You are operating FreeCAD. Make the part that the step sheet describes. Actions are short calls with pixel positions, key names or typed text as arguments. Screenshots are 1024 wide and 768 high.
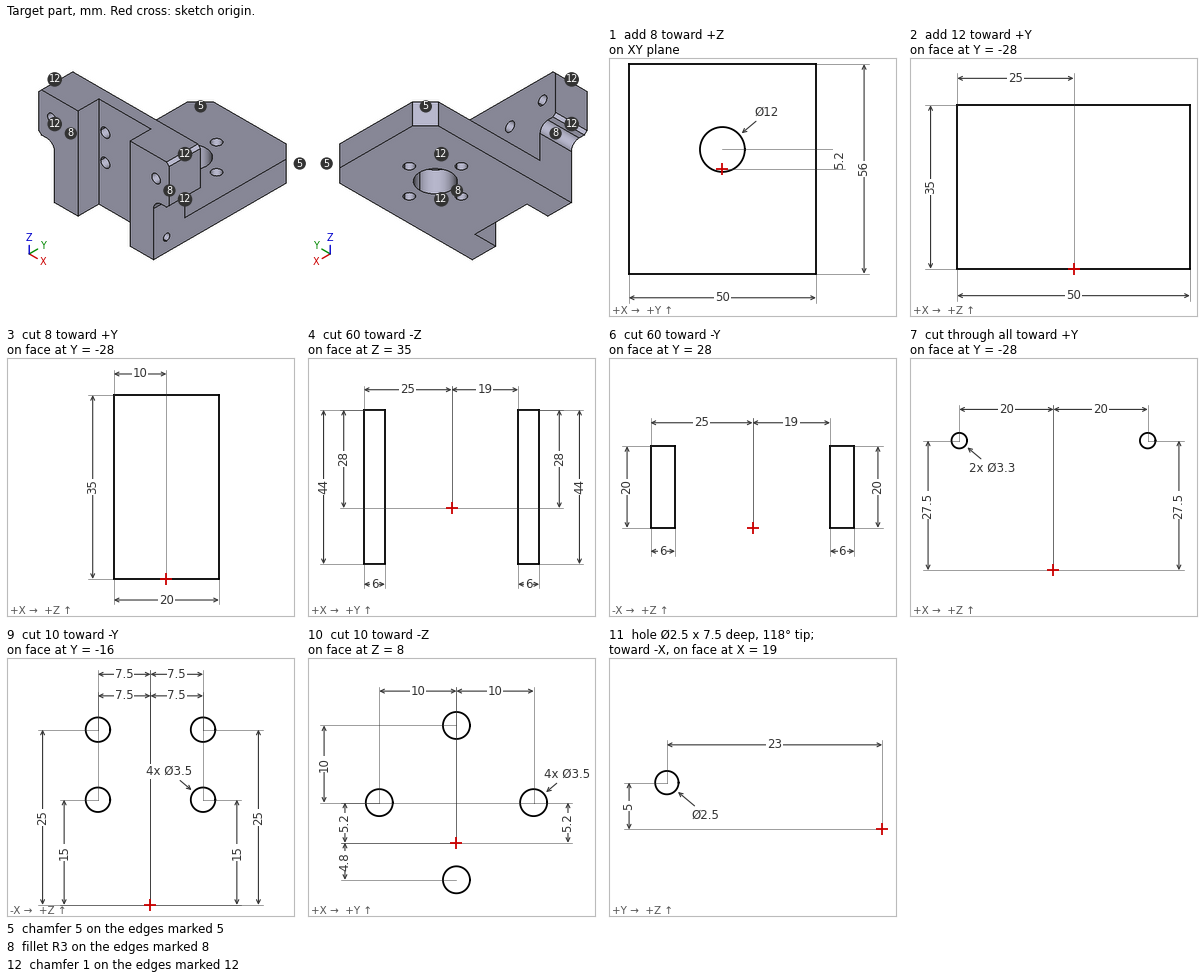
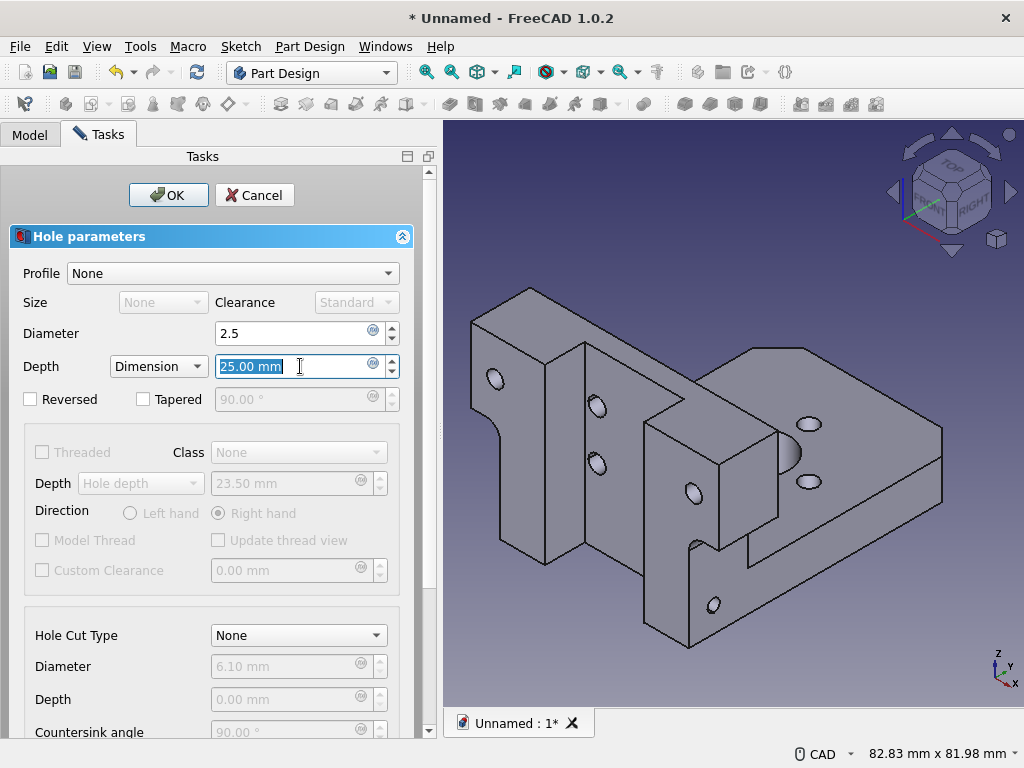
text(7.5)
key(Tab)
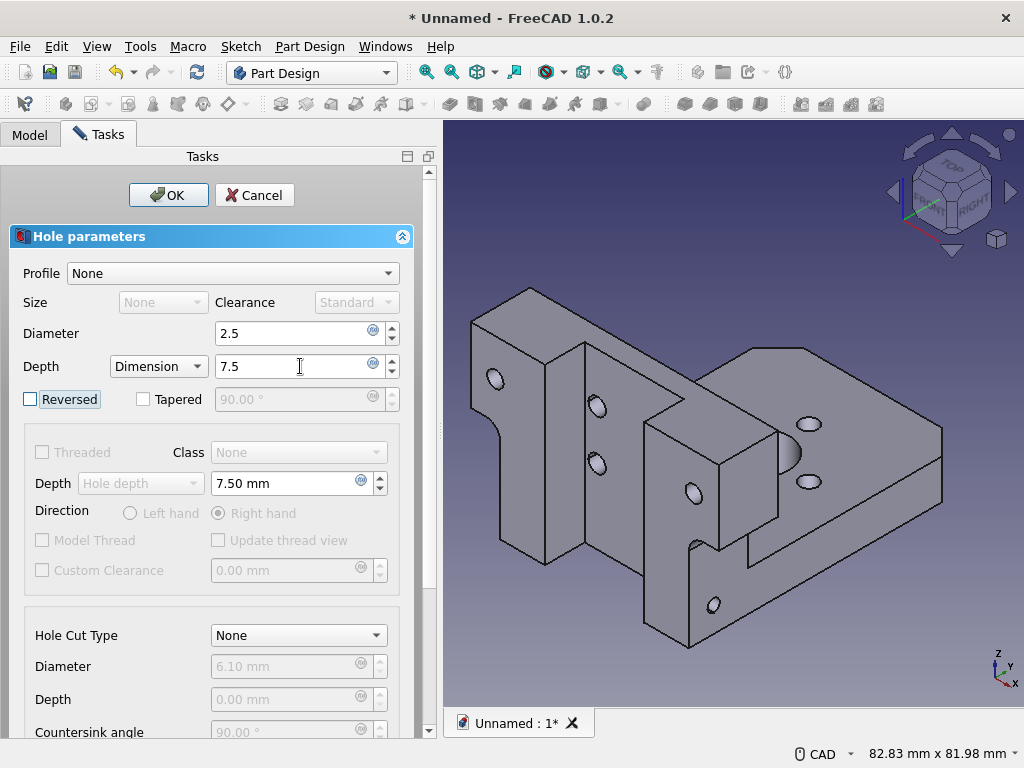
click(169, 195)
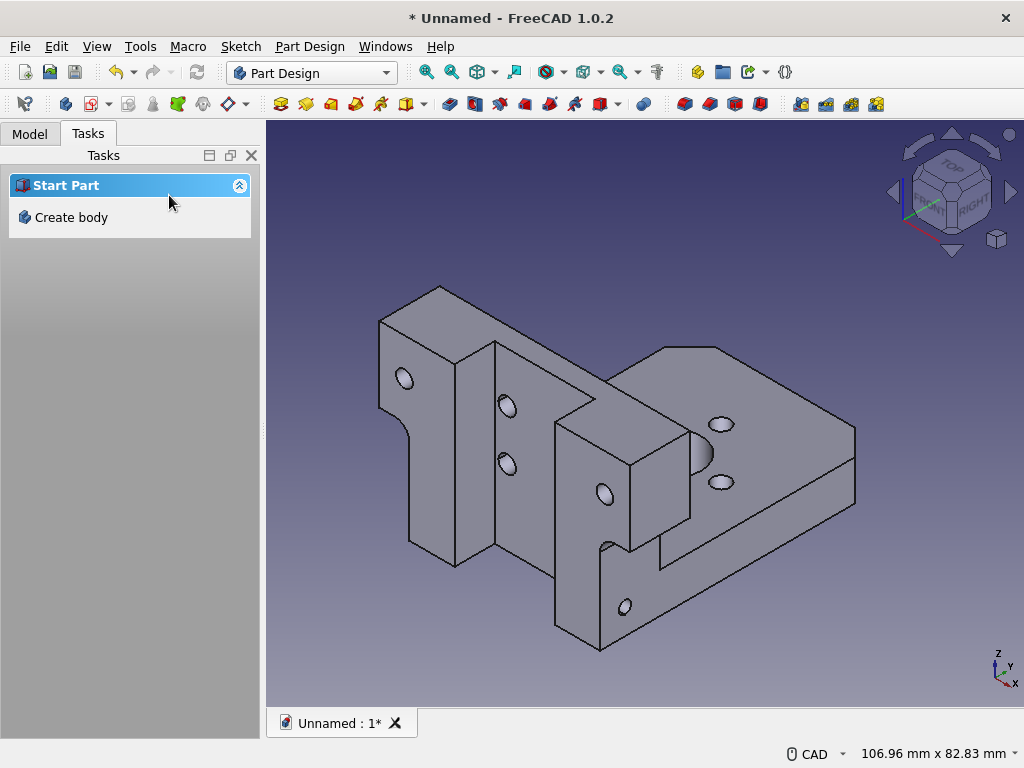
click(660, 447)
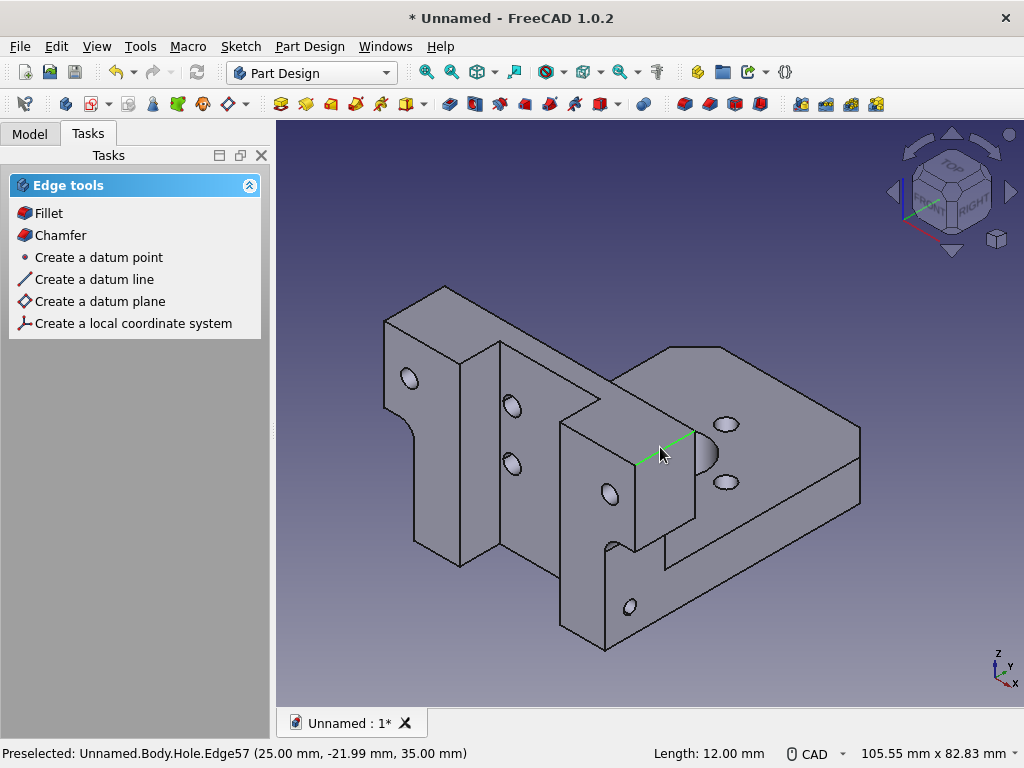
key(2)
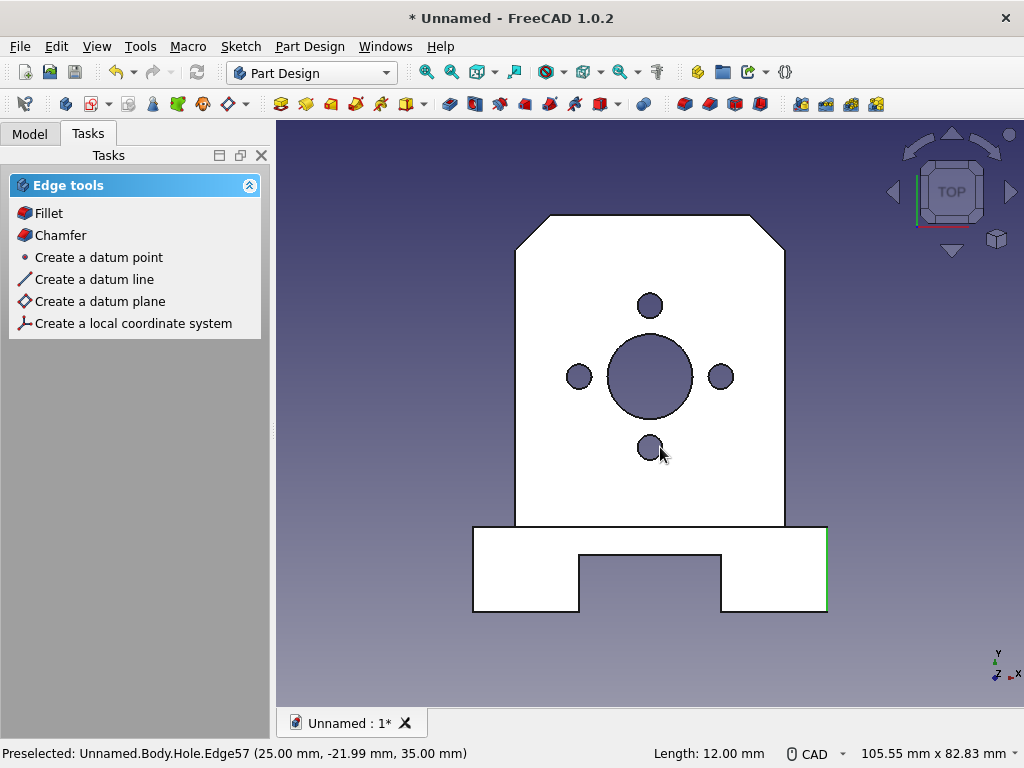
click(473, 568, ctrl)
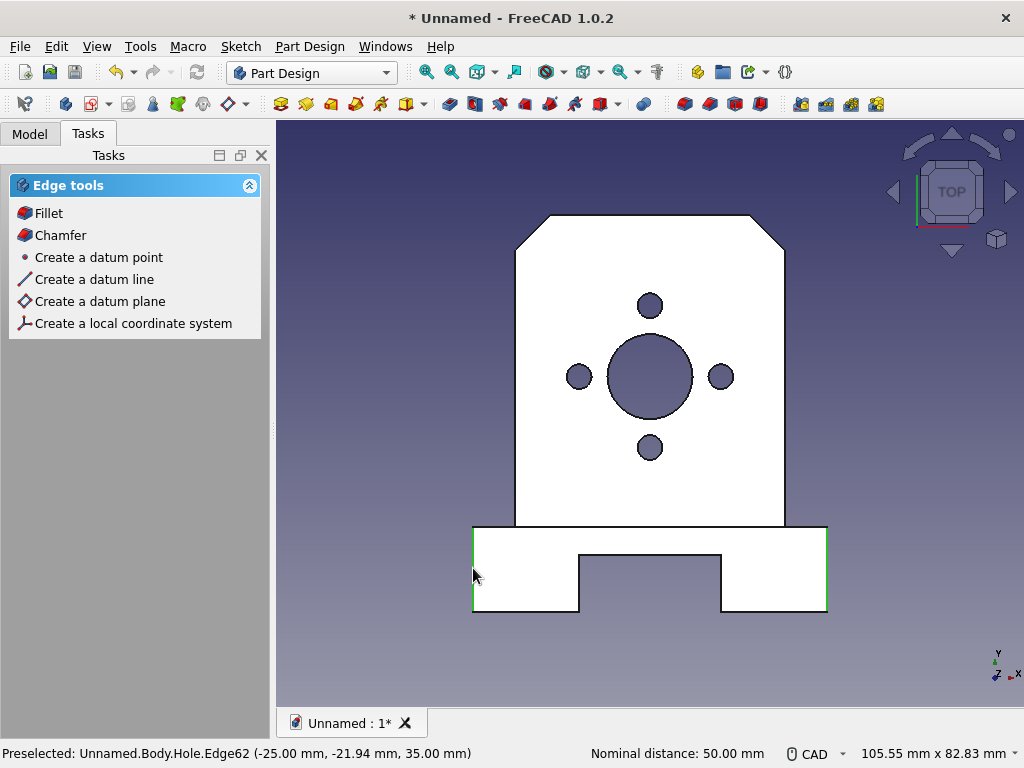
key(0)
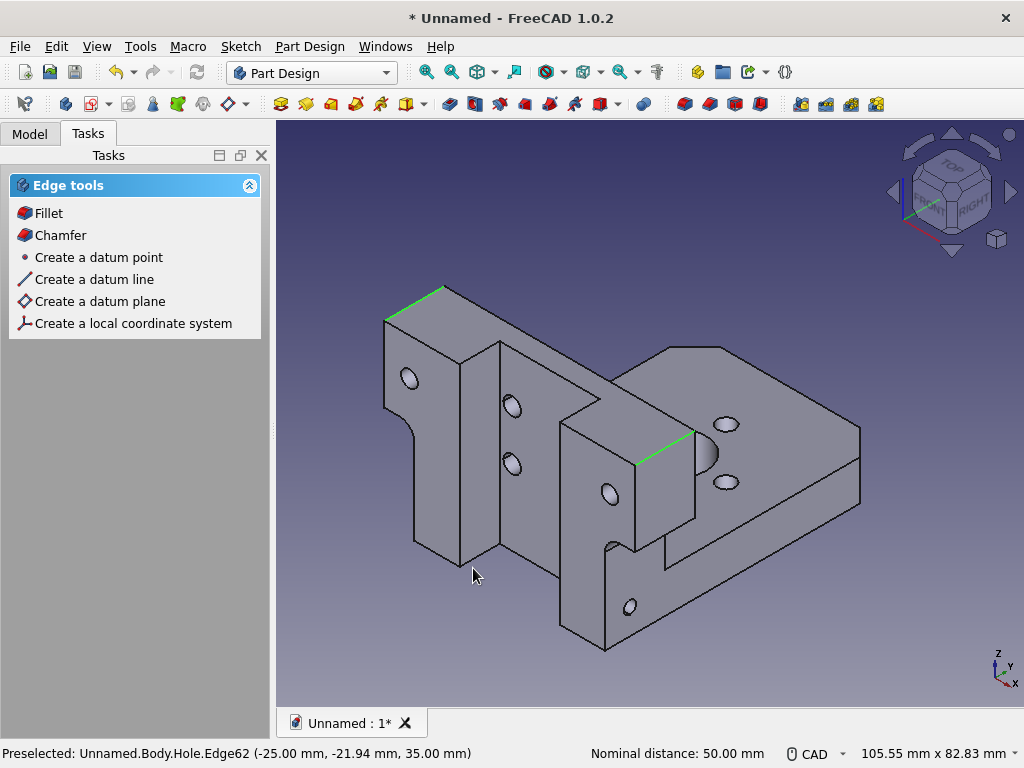
key(1)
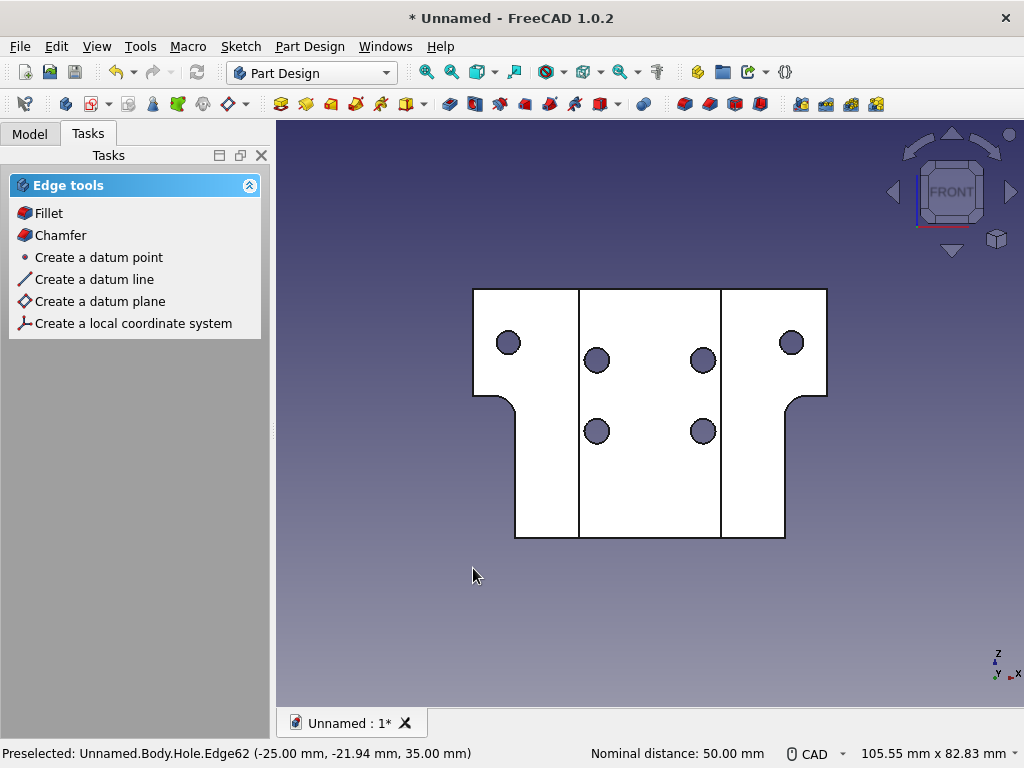
key(3)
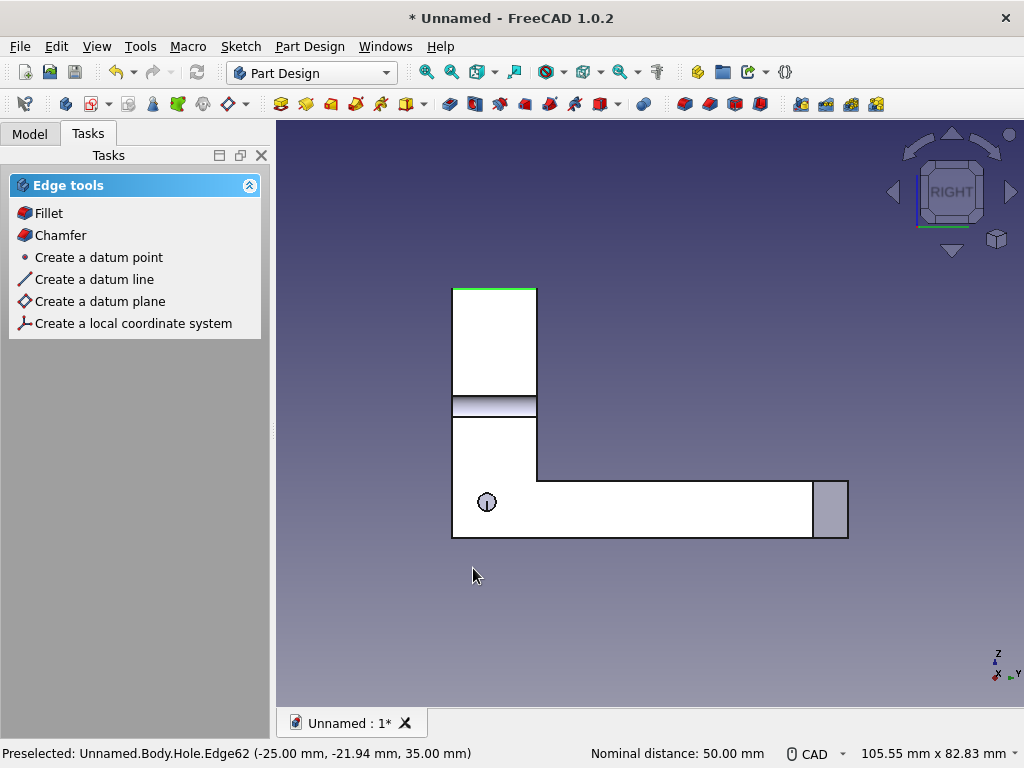
click(494, 395, ctrl)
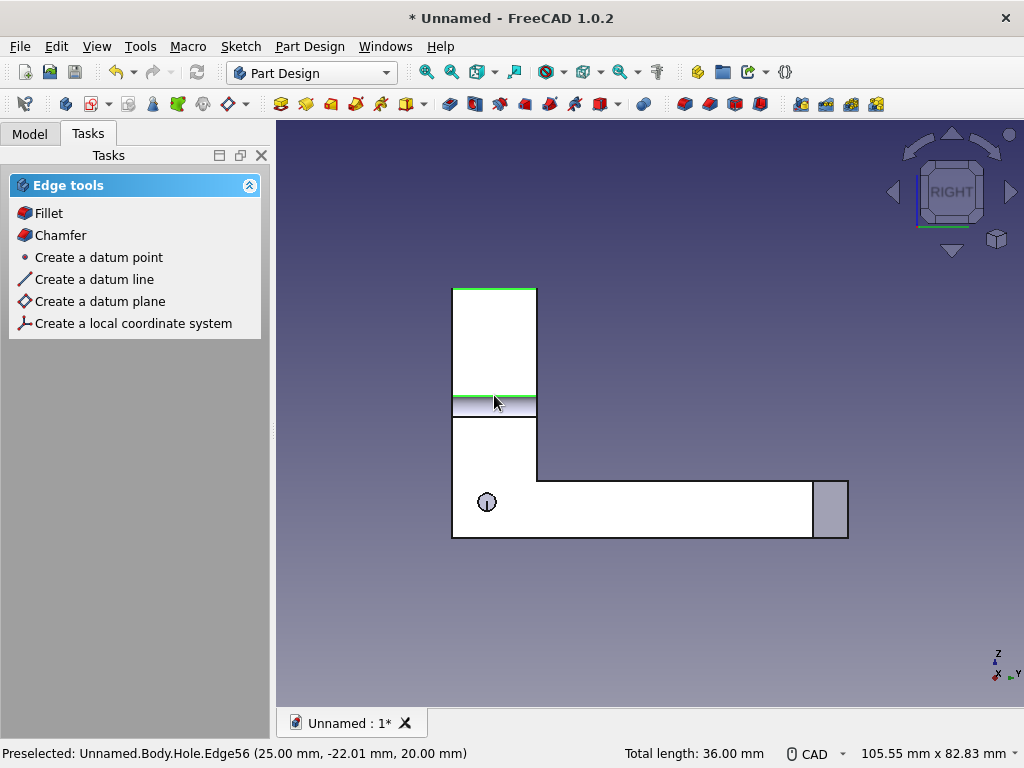
key(5)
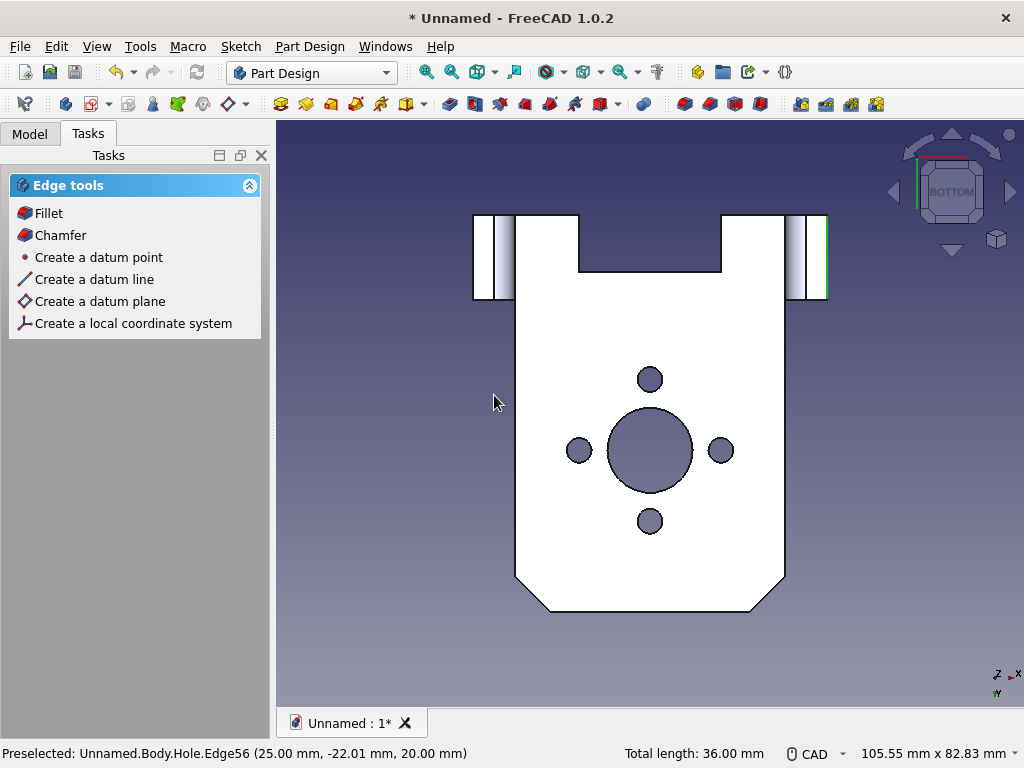
click(473, 257, ctrl)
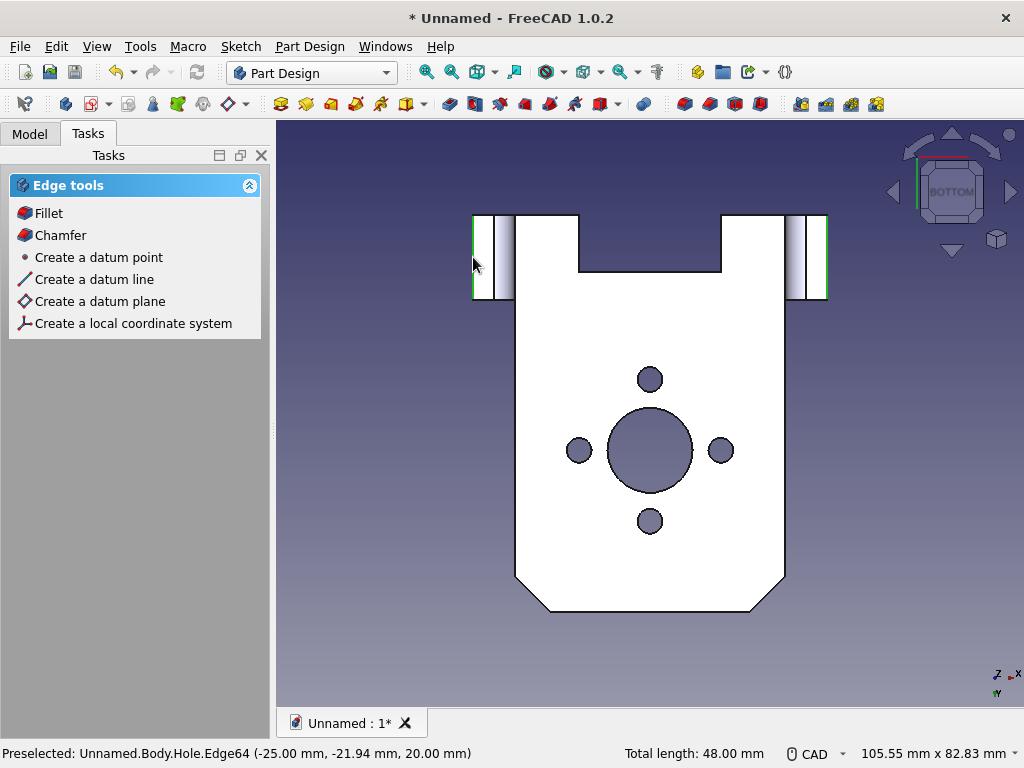
click(710, 104)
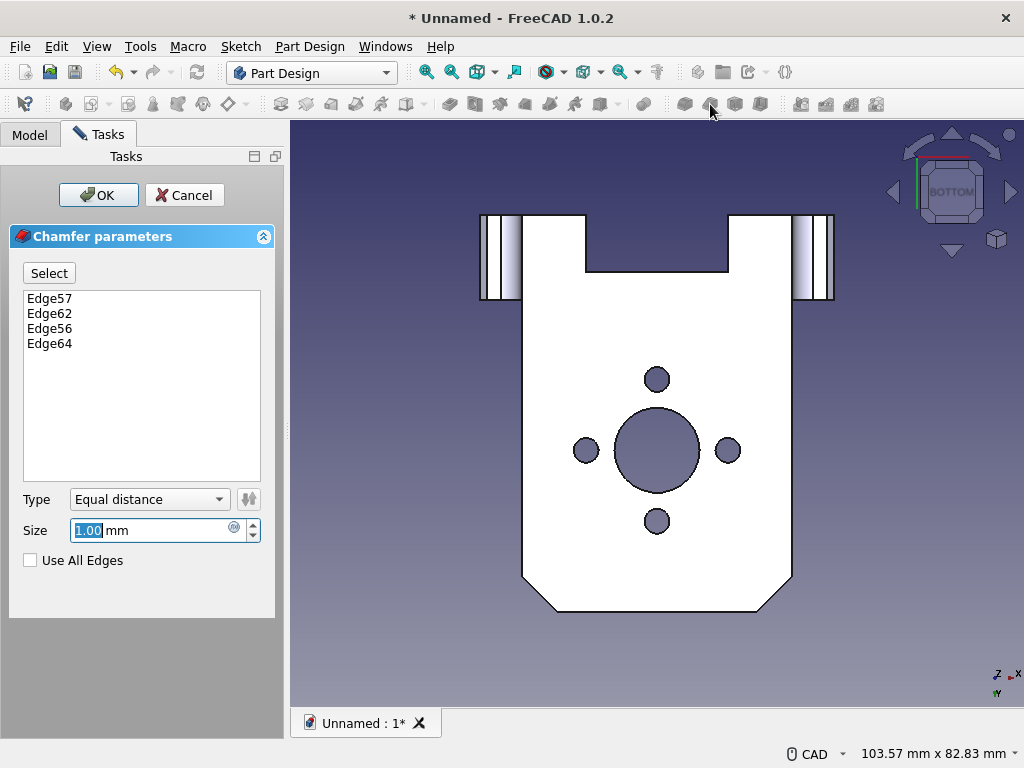
text(1)
key(Tab)